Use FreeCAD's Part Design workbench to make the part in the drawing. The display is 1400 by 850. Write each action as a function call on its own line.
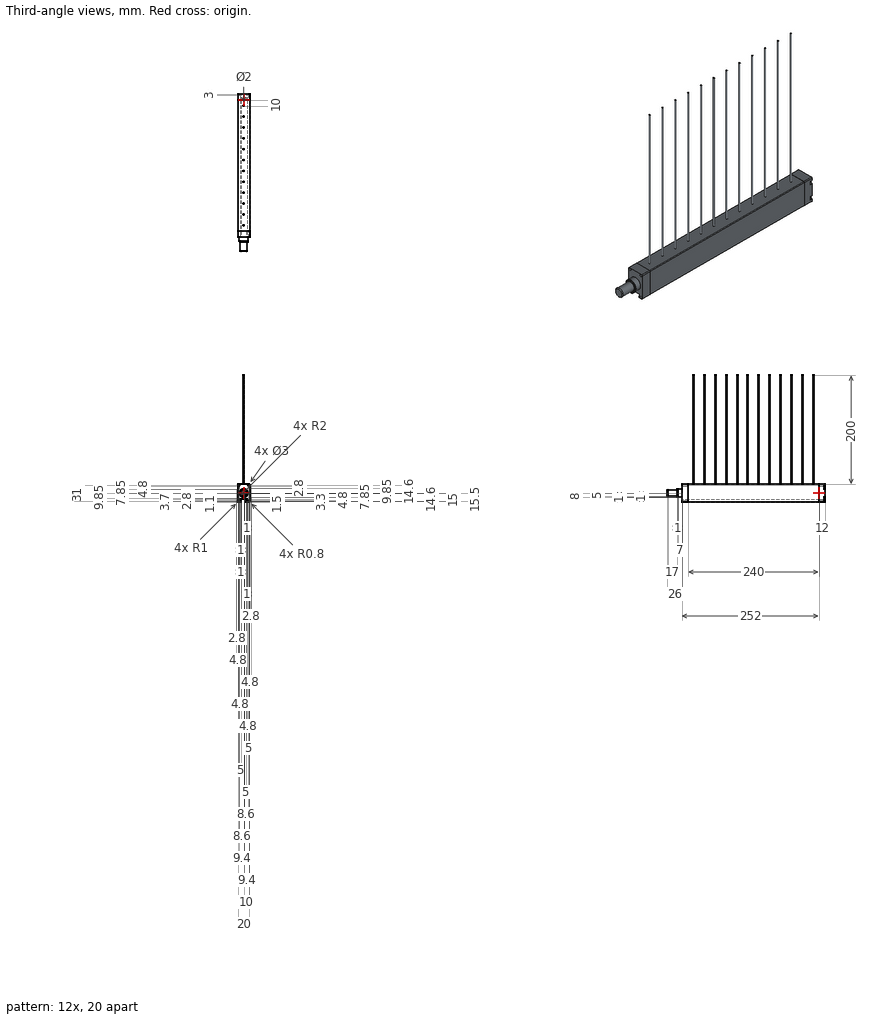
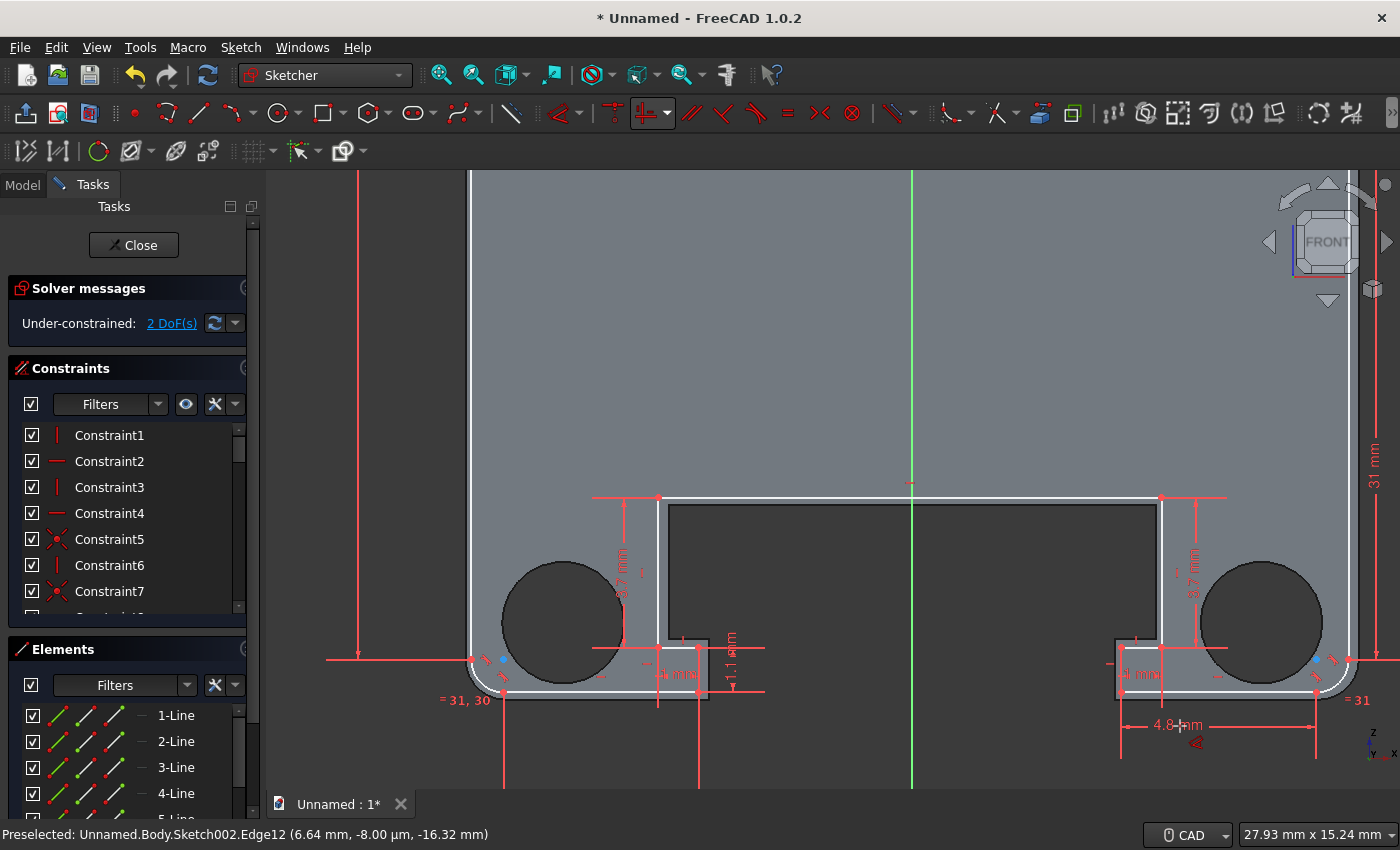
scroll(701, 673, down, 6)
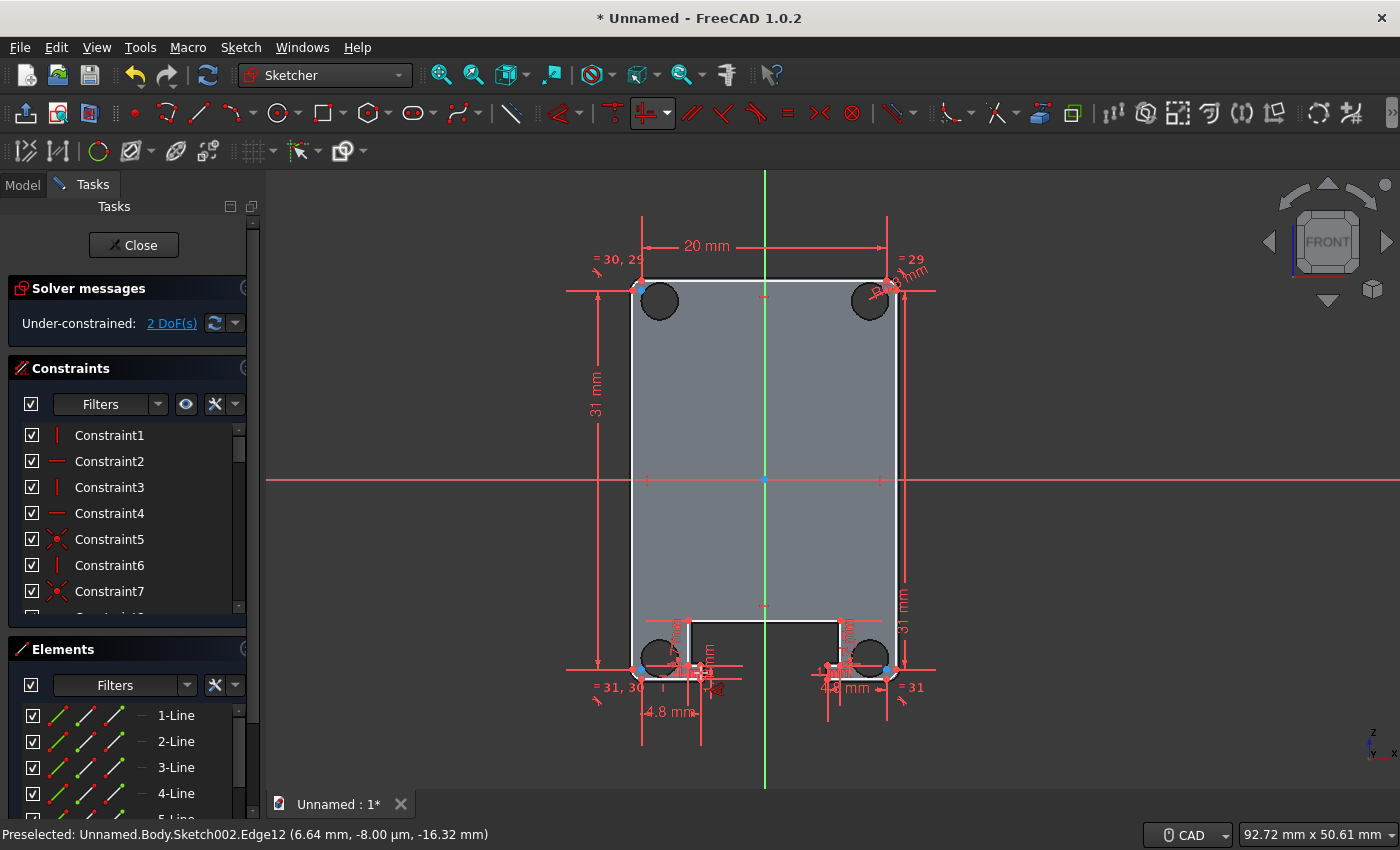
scroll(887, 281, up, 2)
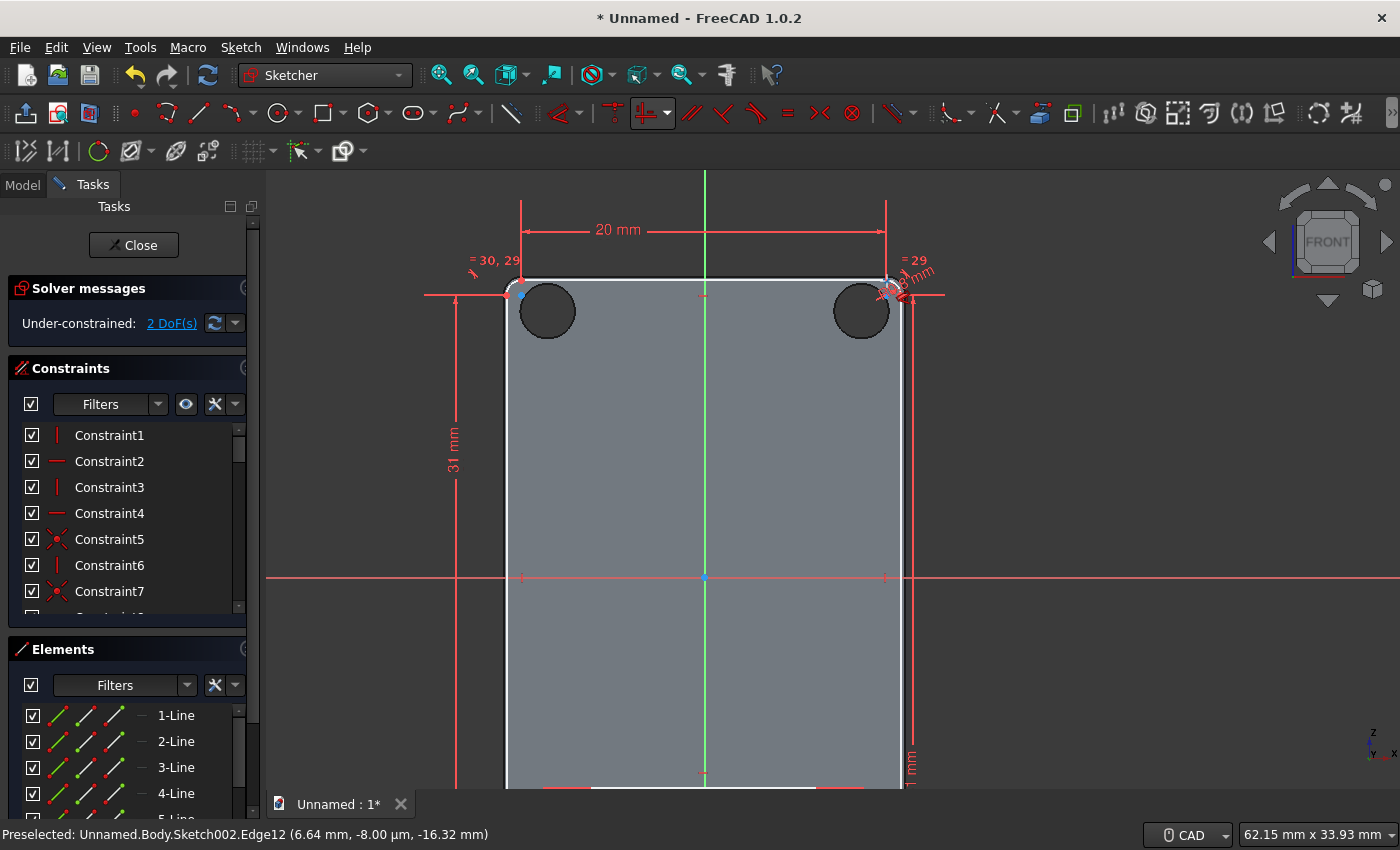
click(886, 280)
click(795, 246)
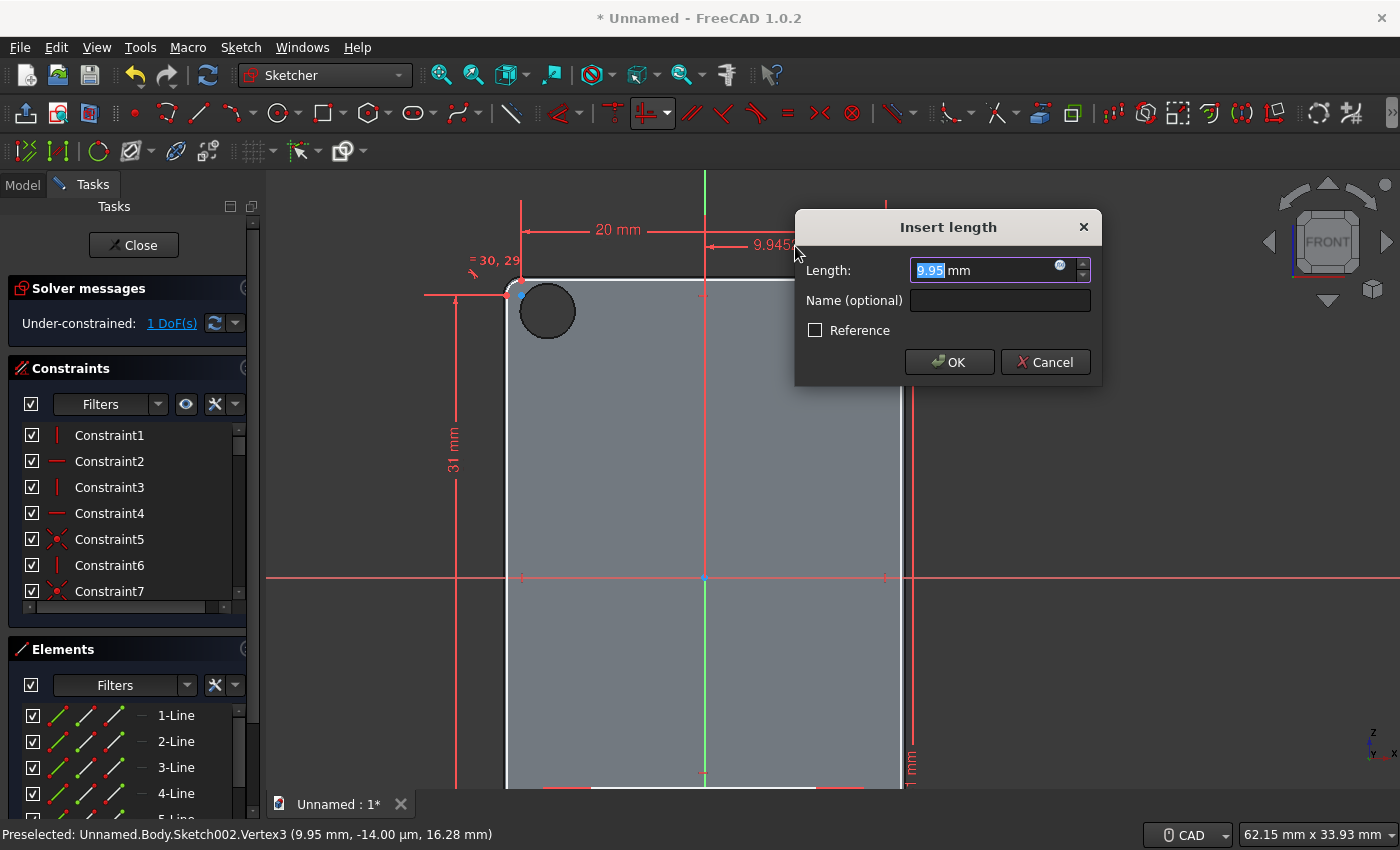
text(10)
key(Return)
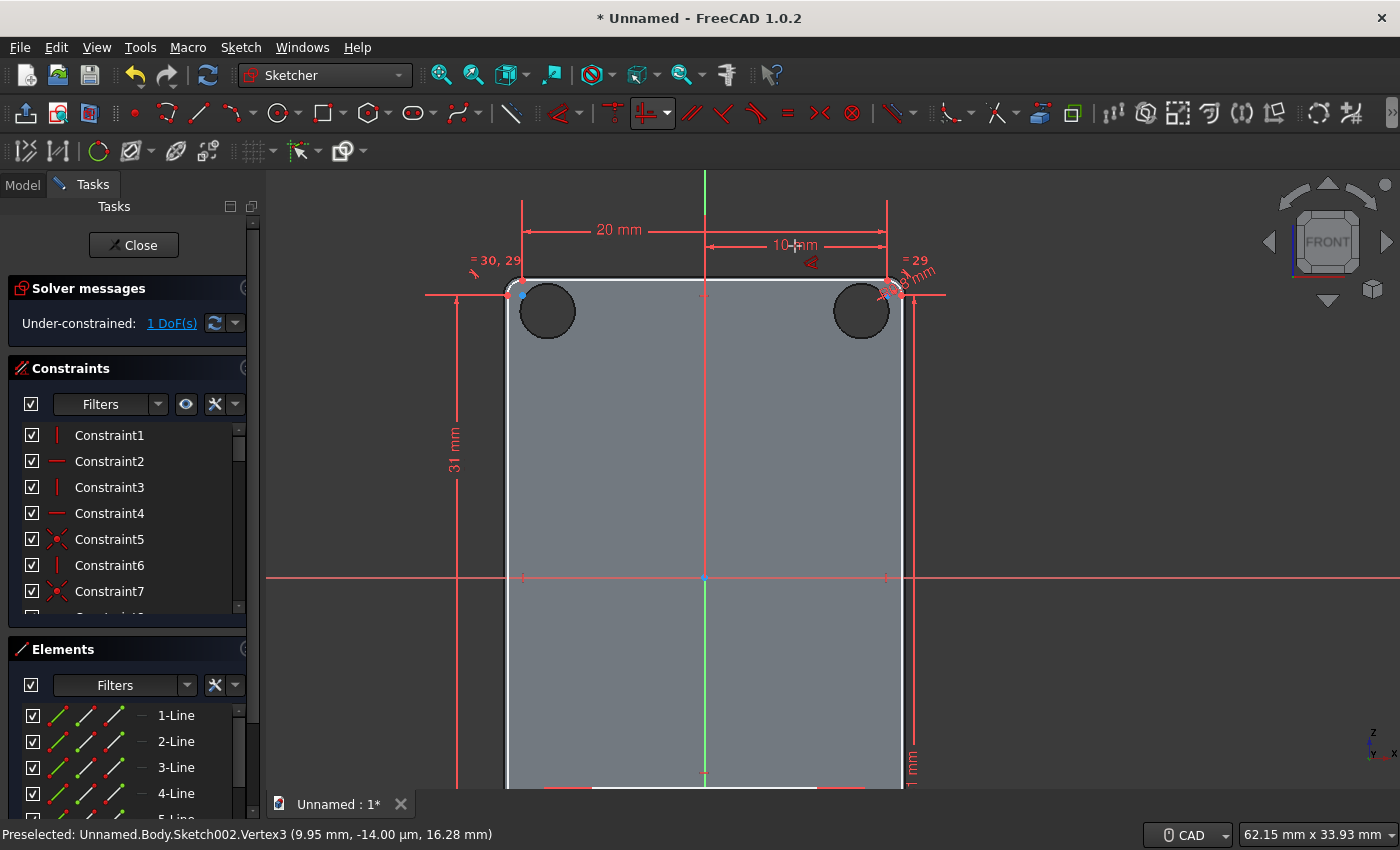
scroll(886, 280, down, 2)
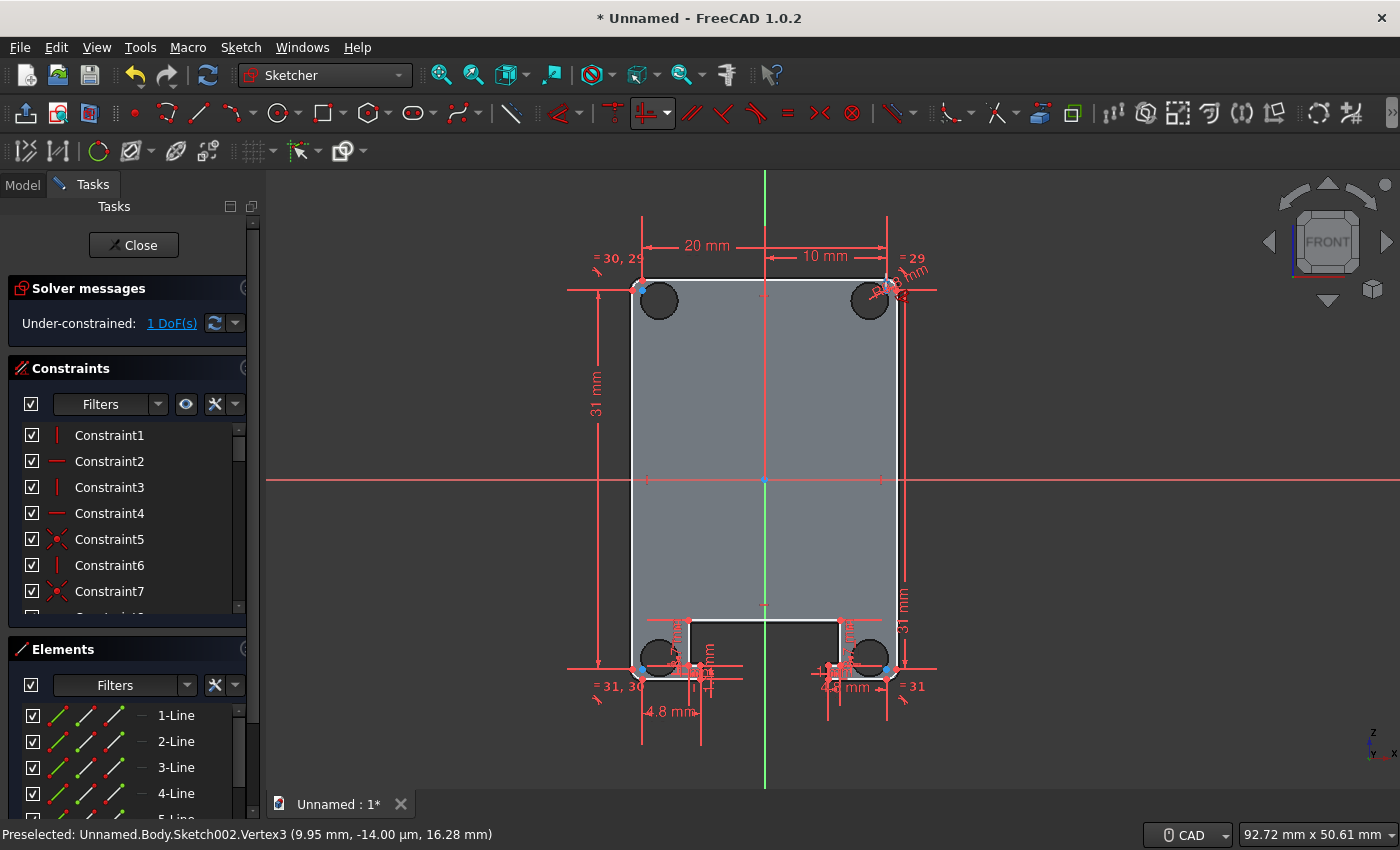
scroll(897, 669, up, 2)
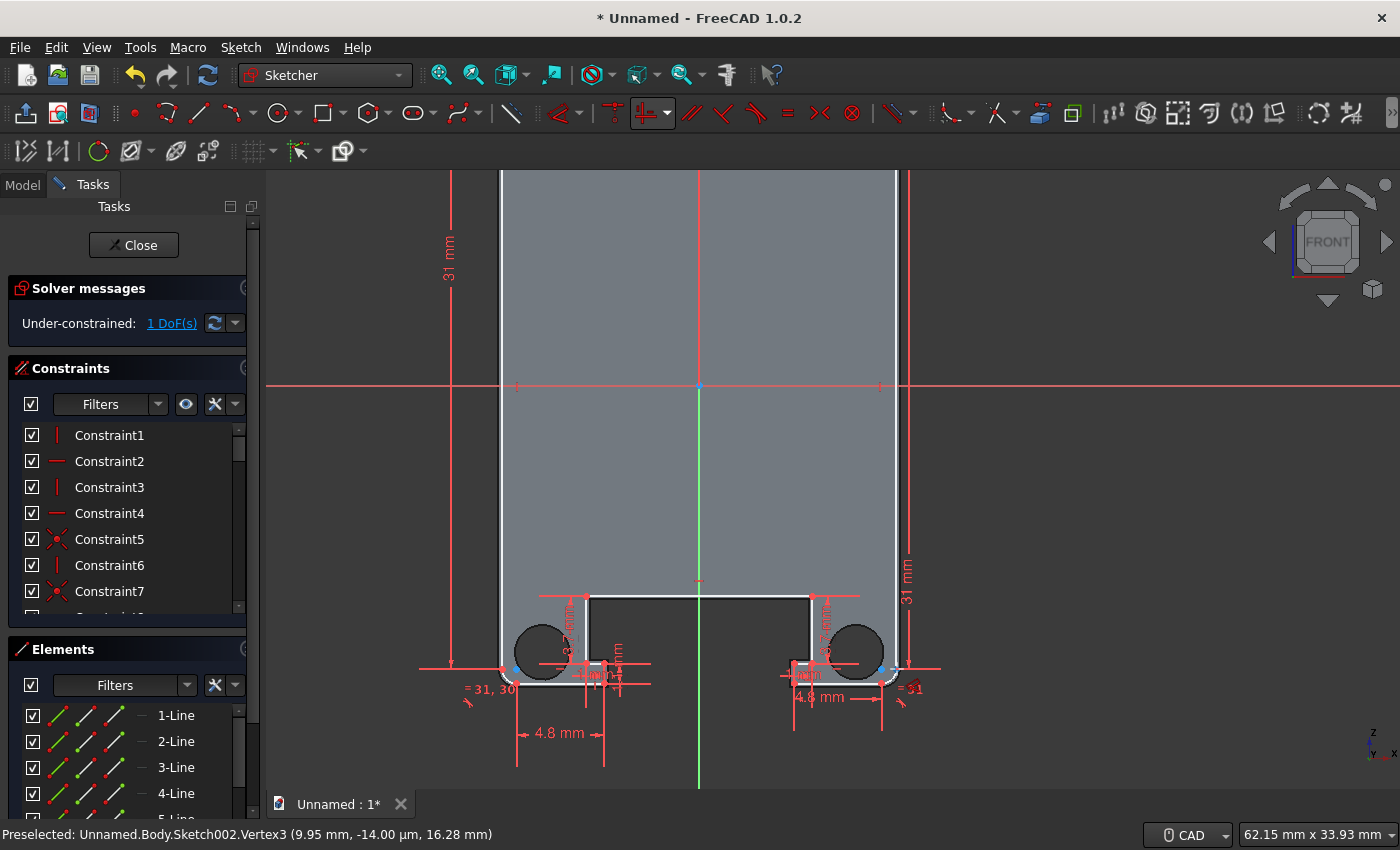
click(896, 669)
click(930, 528)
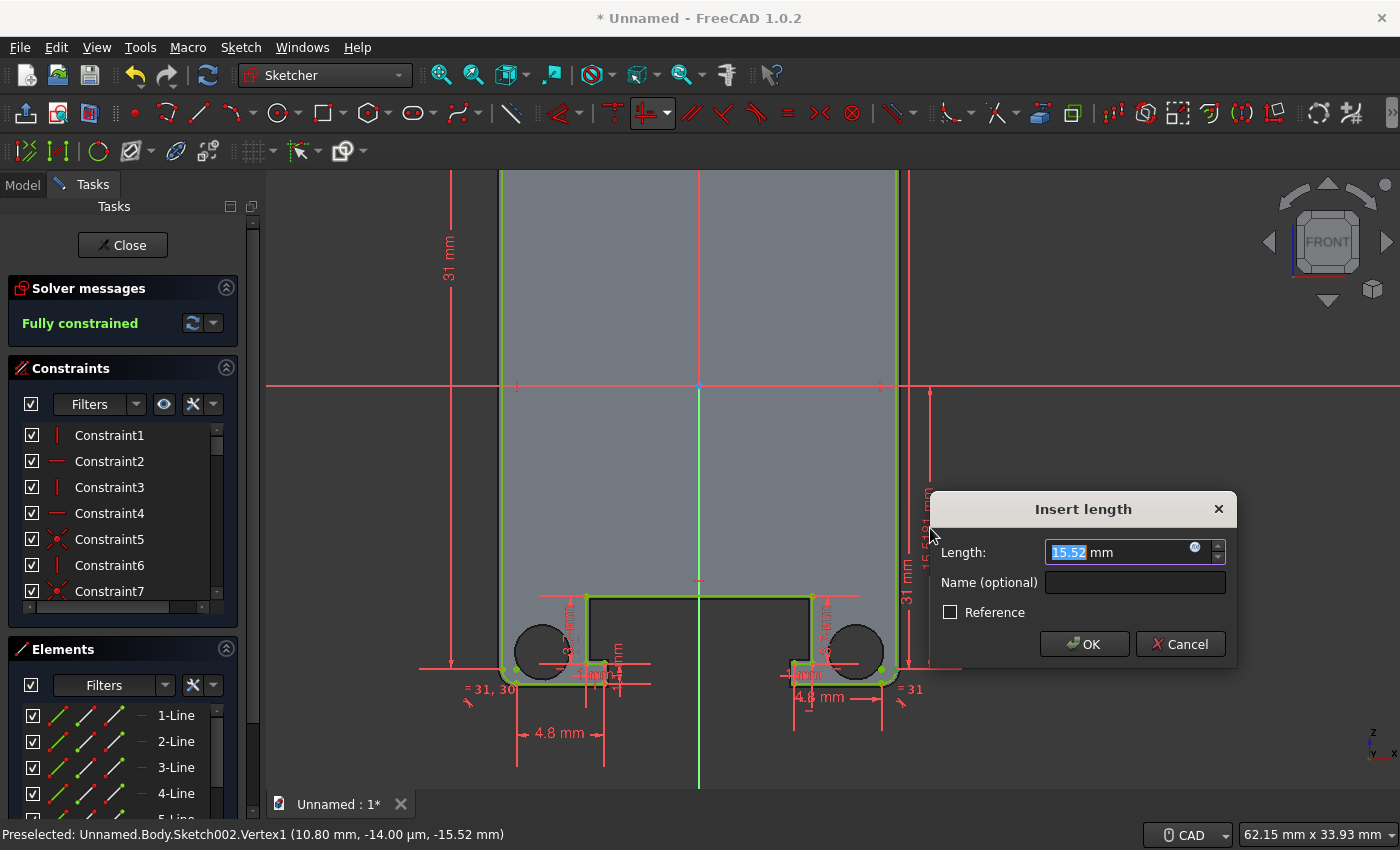
text(15.5)
key(Return)
key(Escape)